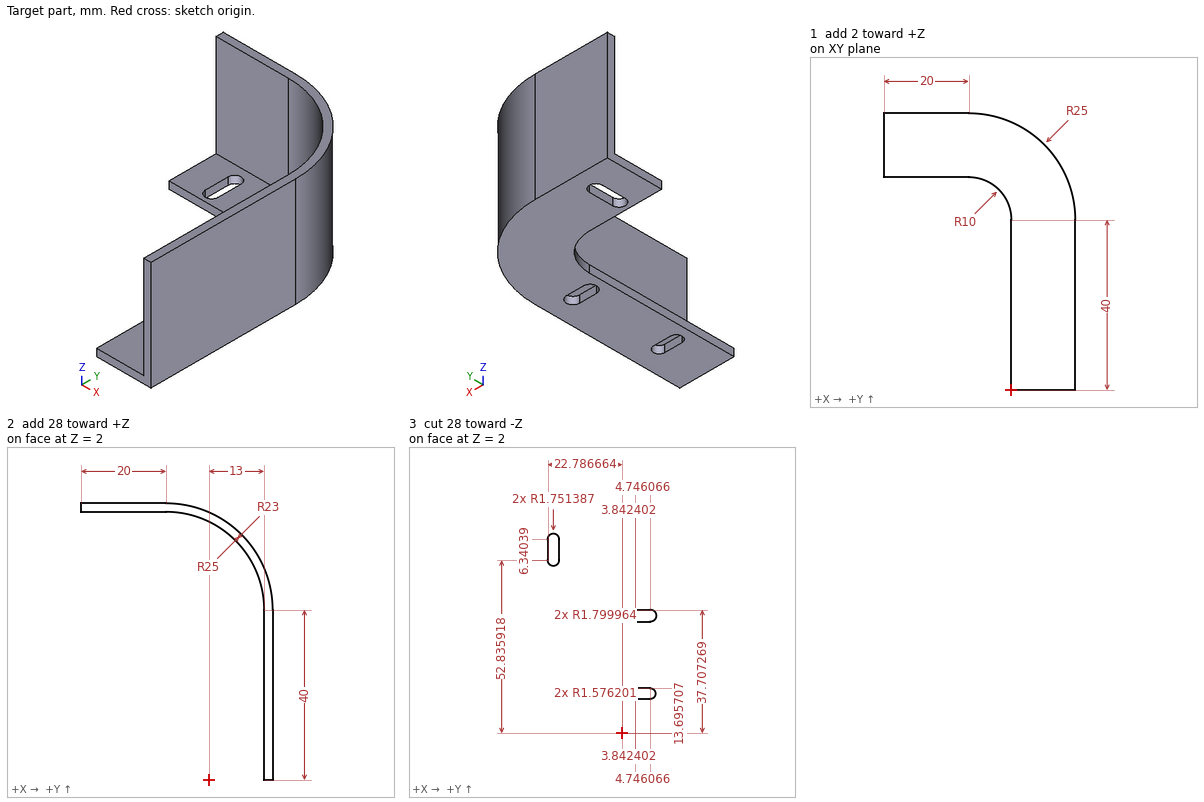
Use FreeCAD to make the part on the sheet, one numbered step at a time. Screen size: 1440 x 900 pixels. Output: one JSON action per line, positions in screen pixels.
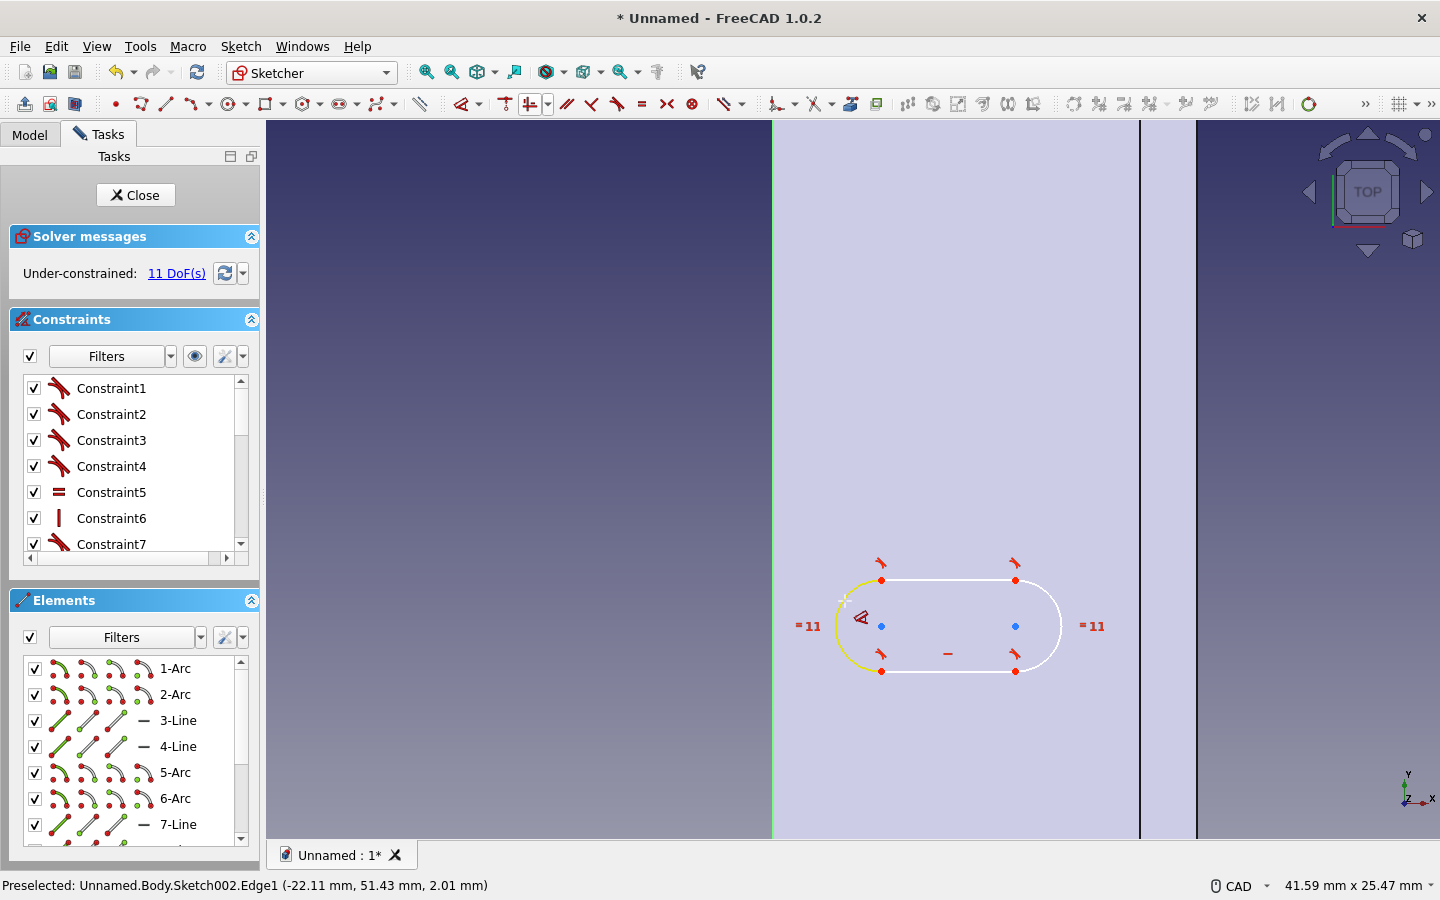
{"action": "left_click", "coordinate": [844, 599]}
{"action": "left_click", "coordinate": [818, 580]}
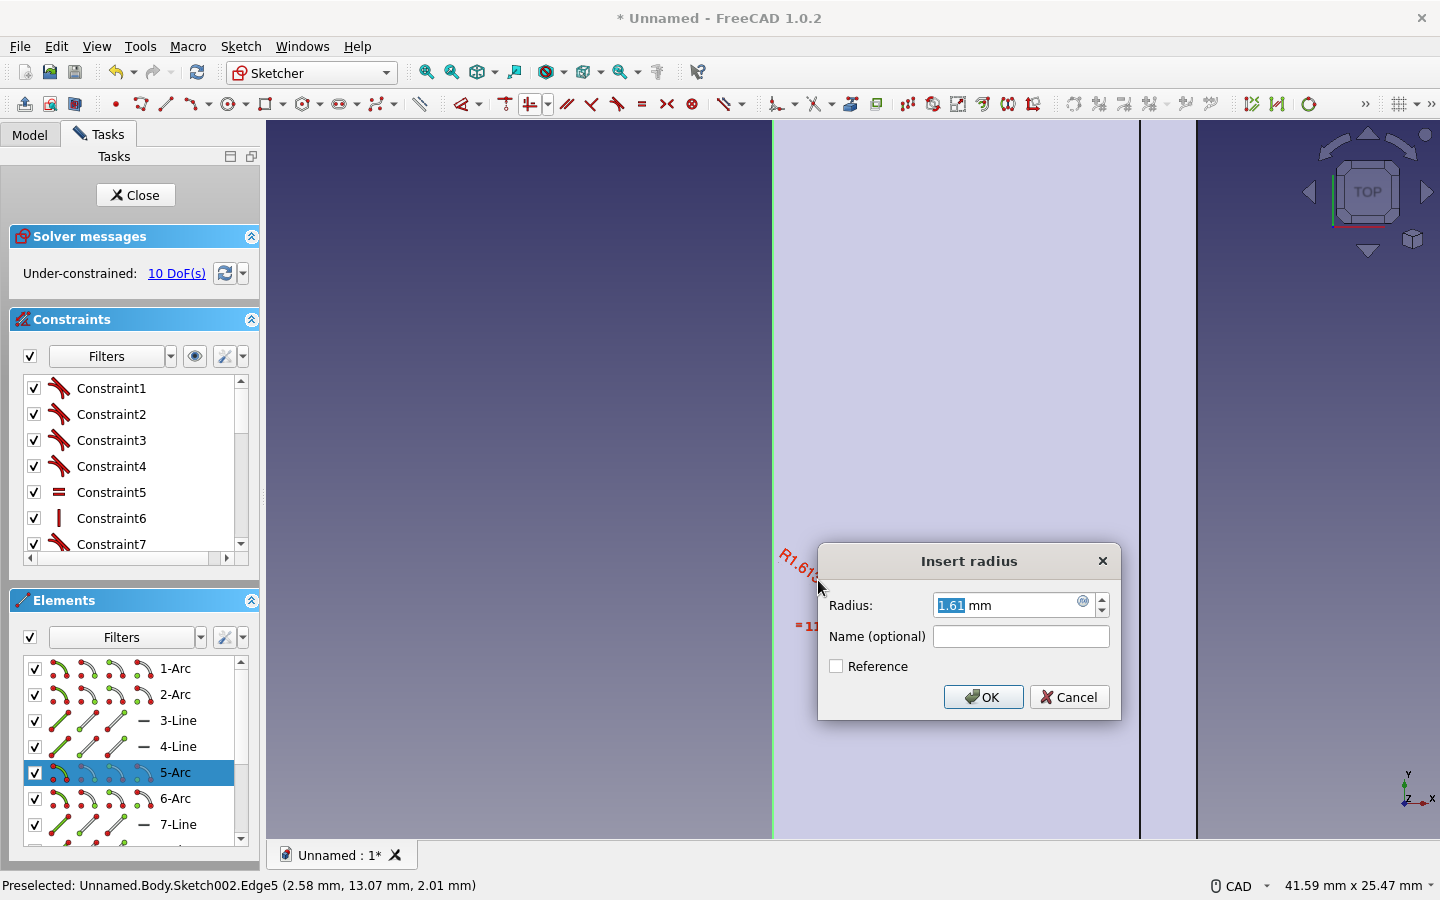
{"action": "type", "text": "1.576201"}
{"action": "key", "text": "Return"}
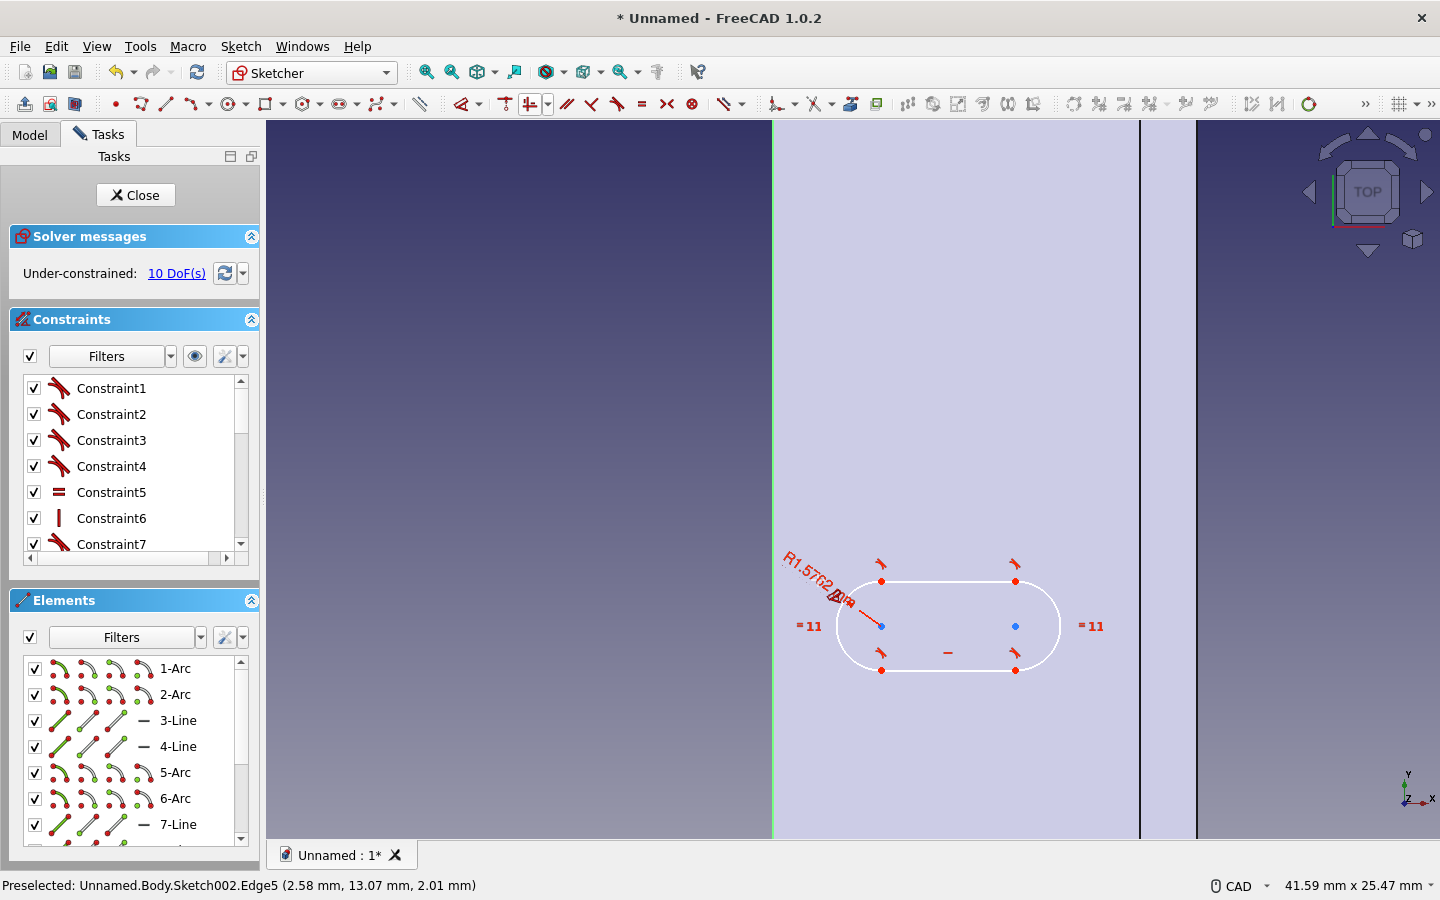
{"action": "scroll", "coordinate": [845, 602], "scroll_direction": "down", "scroll_amount": 7}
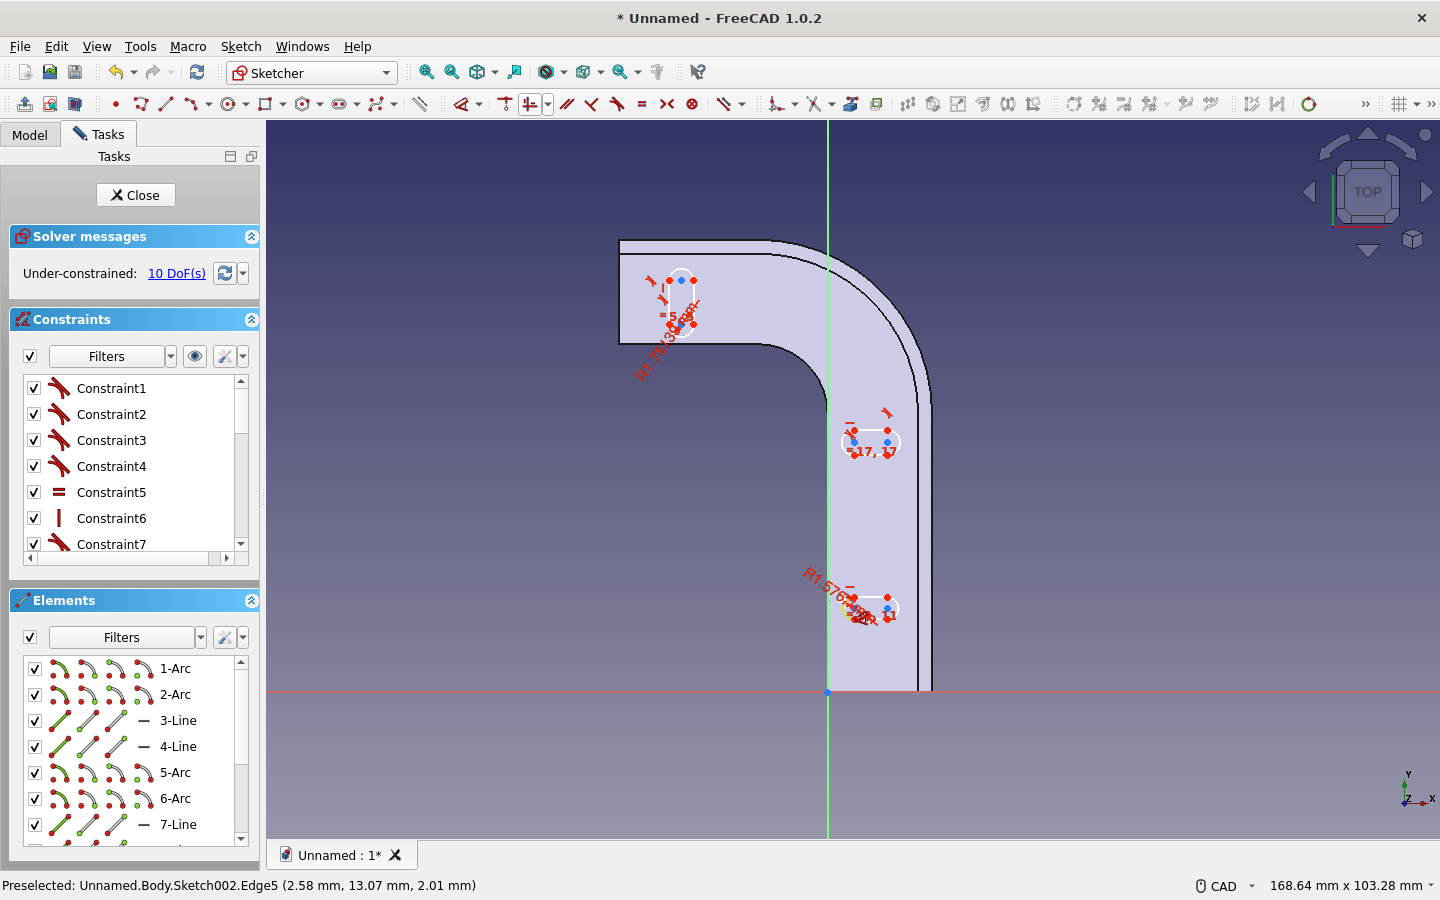
{"action": "scroll", "coordinate": [844, 435], "scroll_direction": "up", "scroll_amount": 6}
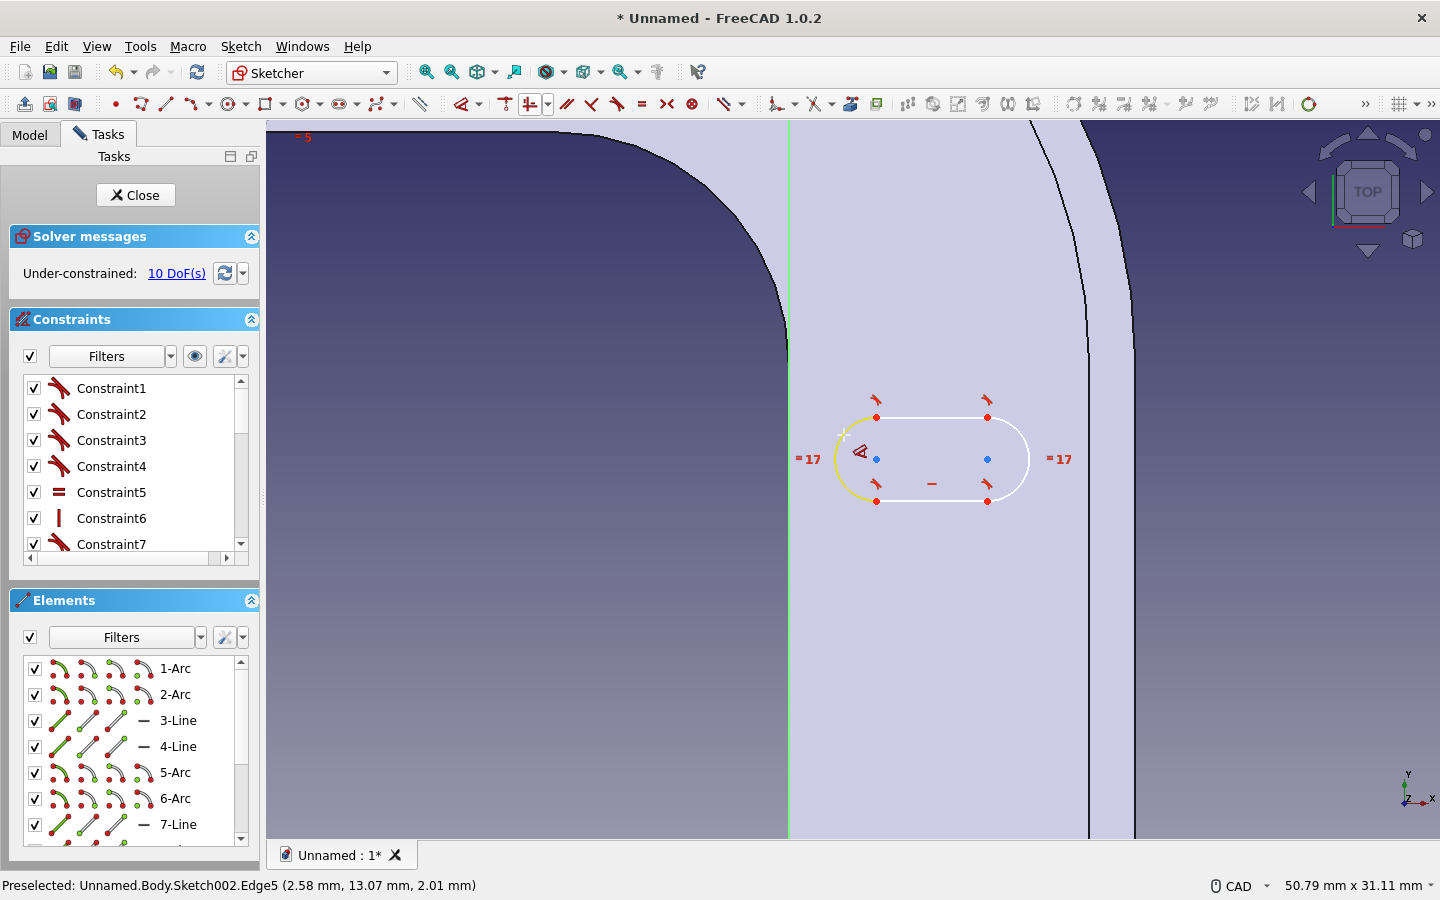
{"action": "left_click", "coordinate": [843, 435]}
{"action": "left_click", "coordinate": [817, 416]}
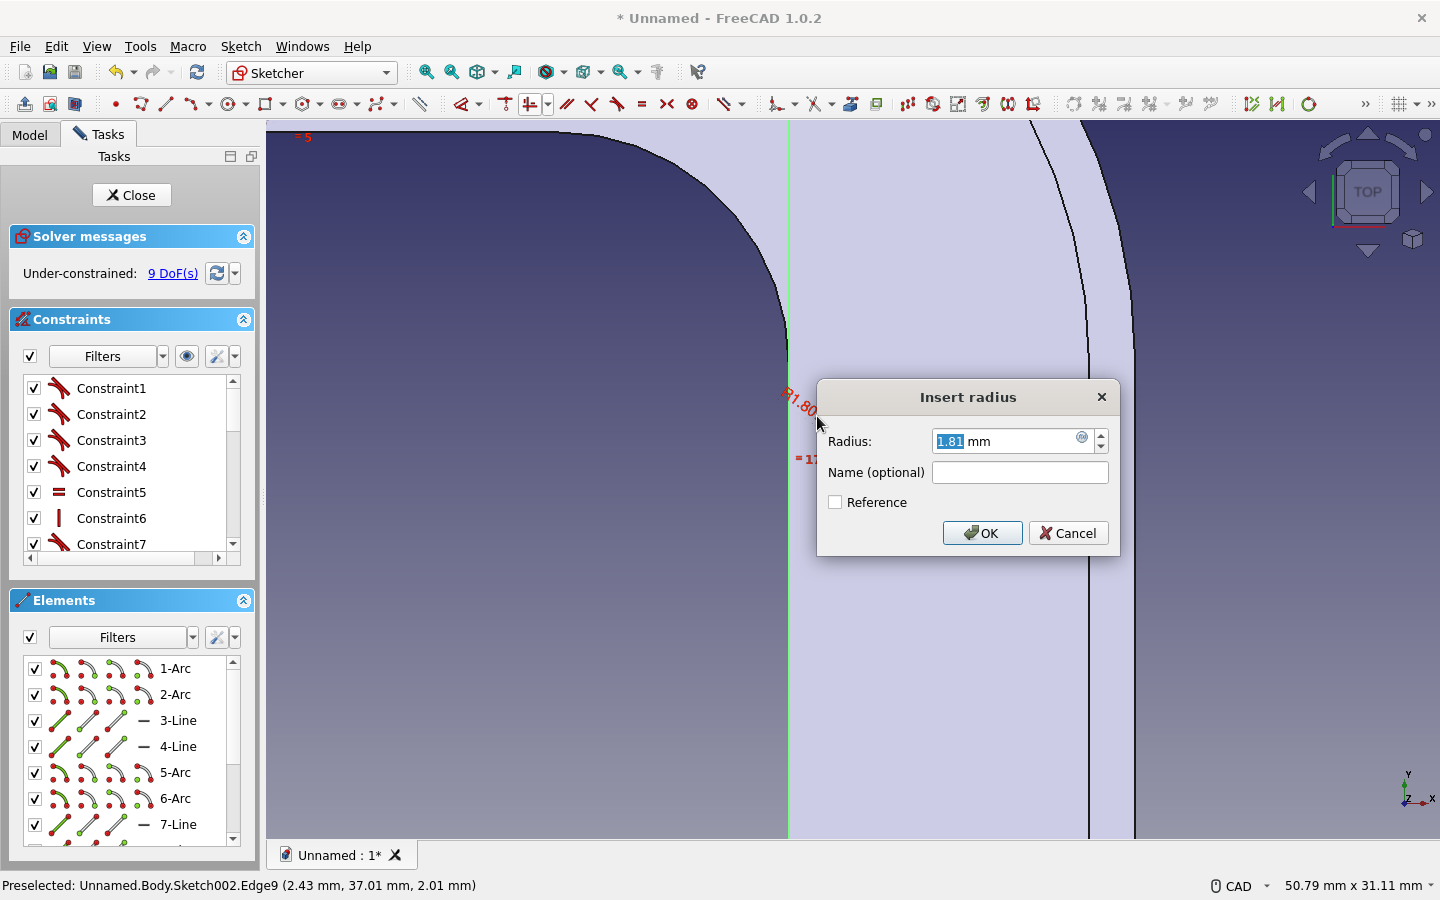
{"action": "type", "text": "1.799964"}
{"action": "key", "text": "Return"}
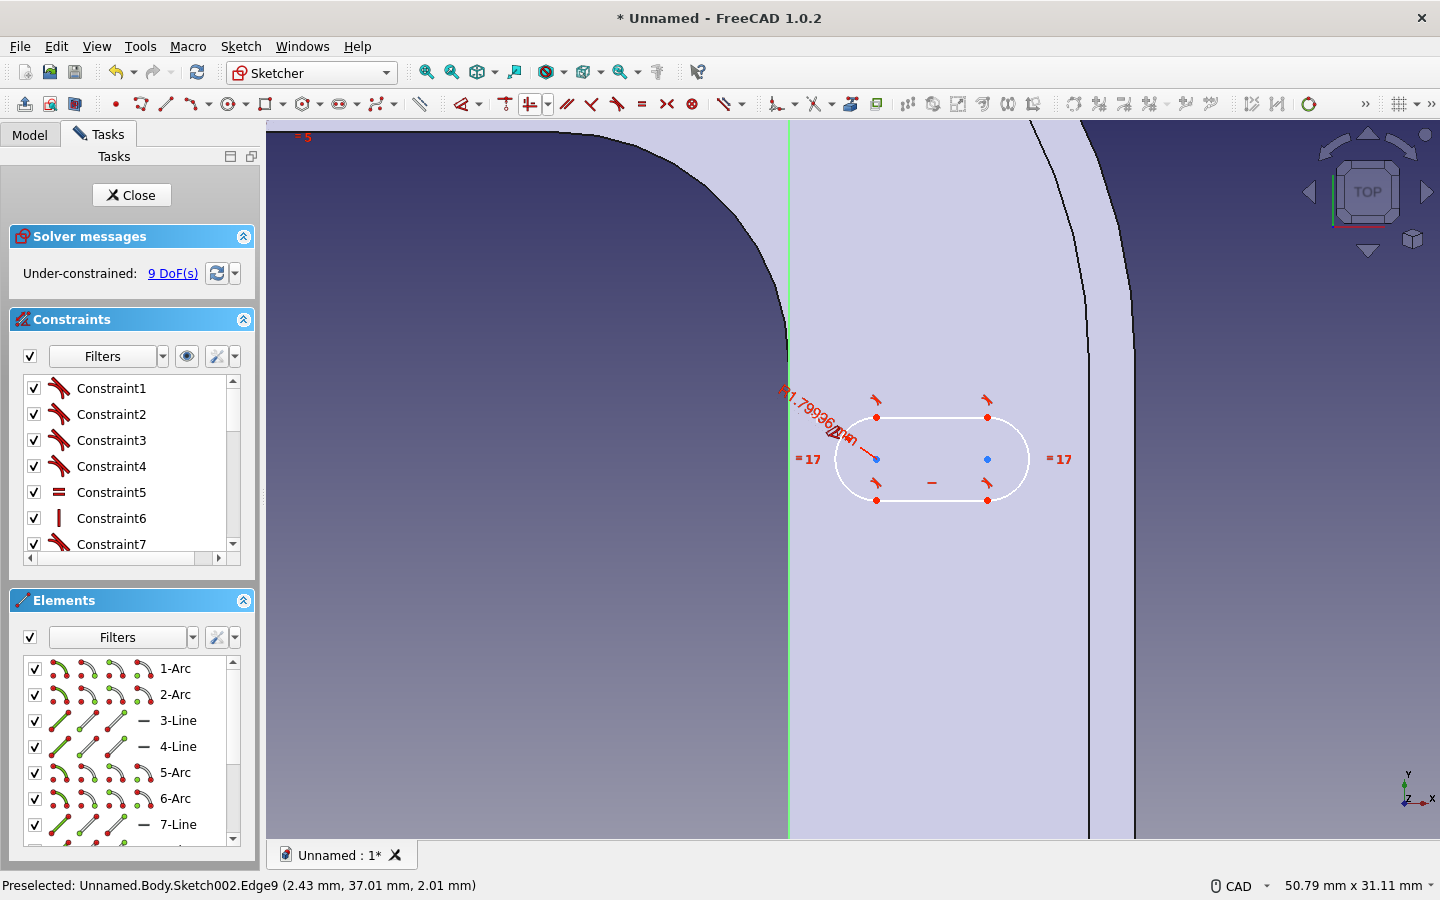
{"action": "scroll", "coordinate": [844, 435], "scroll_direction": "down", "scroll_amount": 6}